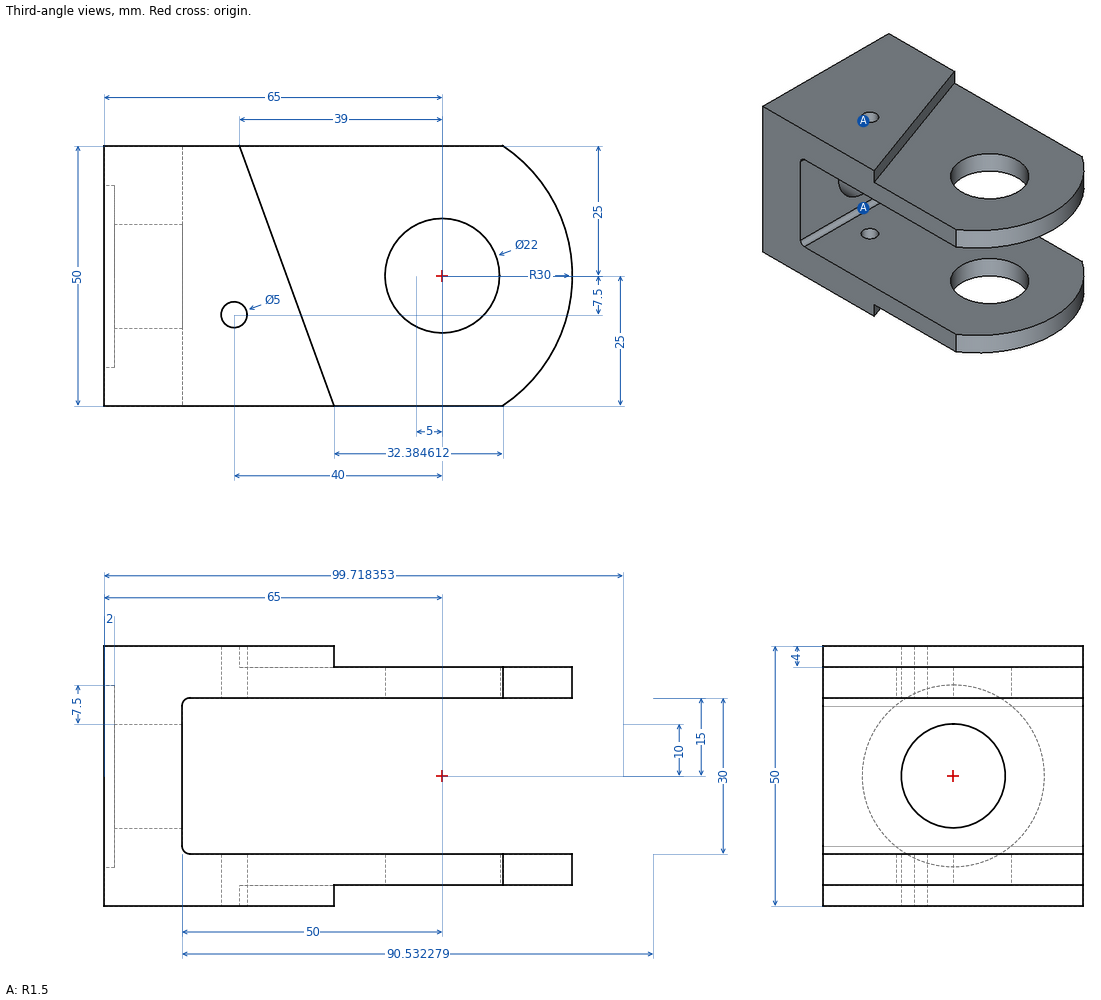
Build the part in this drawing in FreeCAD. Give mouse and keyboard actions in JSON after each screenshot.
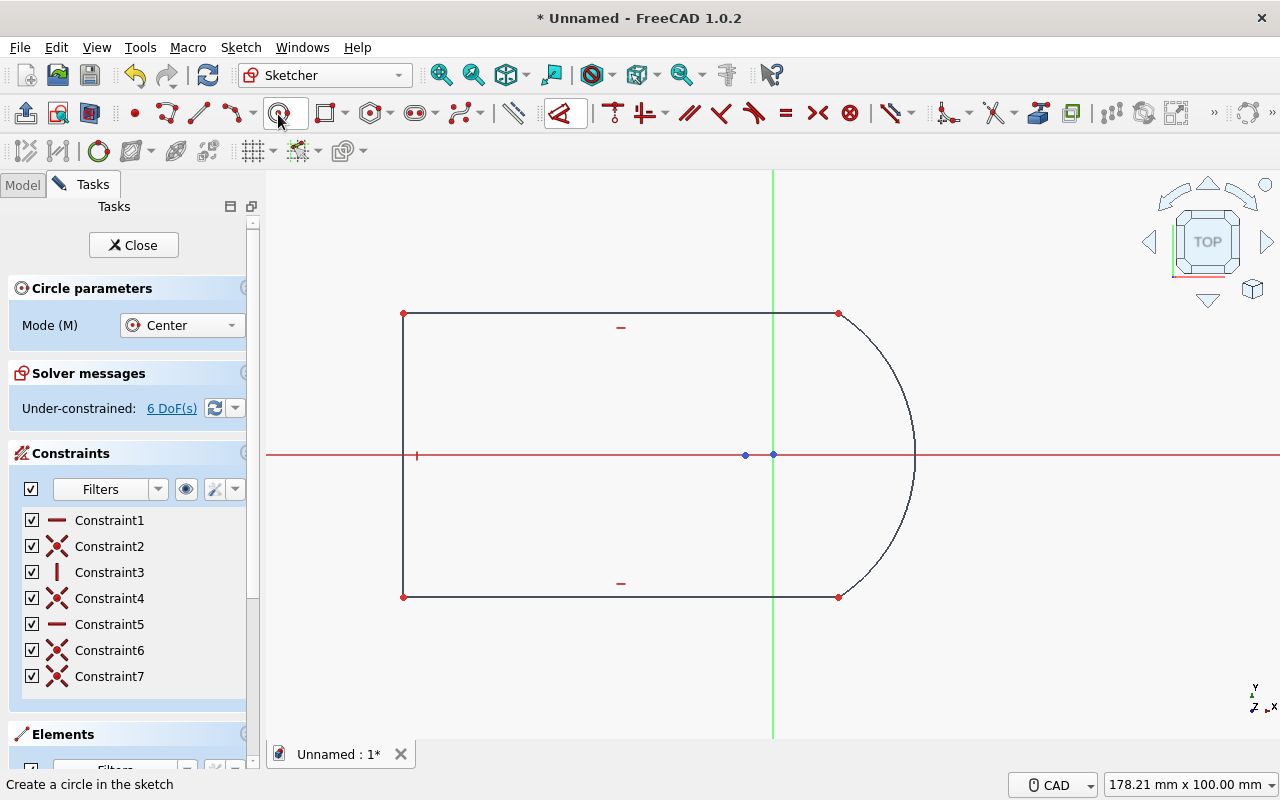
{"action": "scroll", "coordinate": [545, 497], "scroll_direction": "up", "scroll_amount": 3}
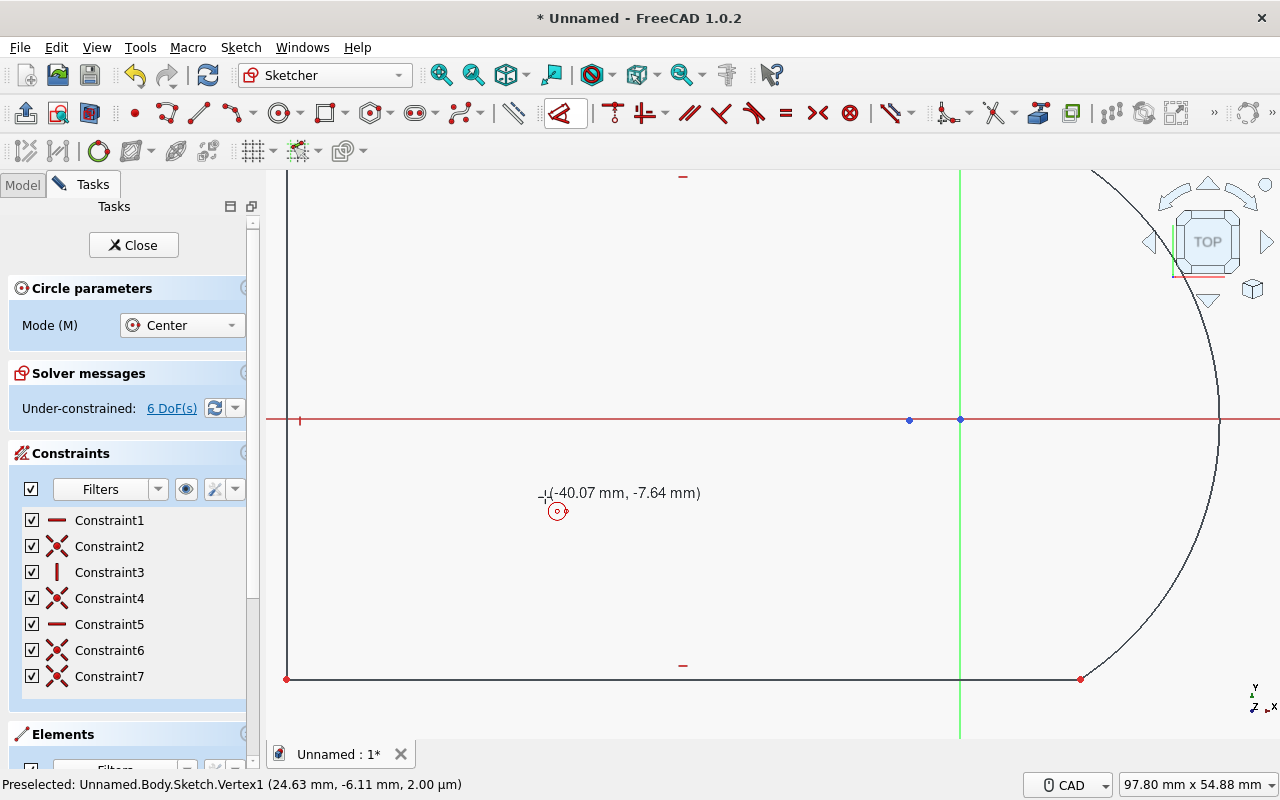
{"action": "left_click", "coordinate": [546, 497]}
{"action": "left_click", "coordinate": [564, 479]}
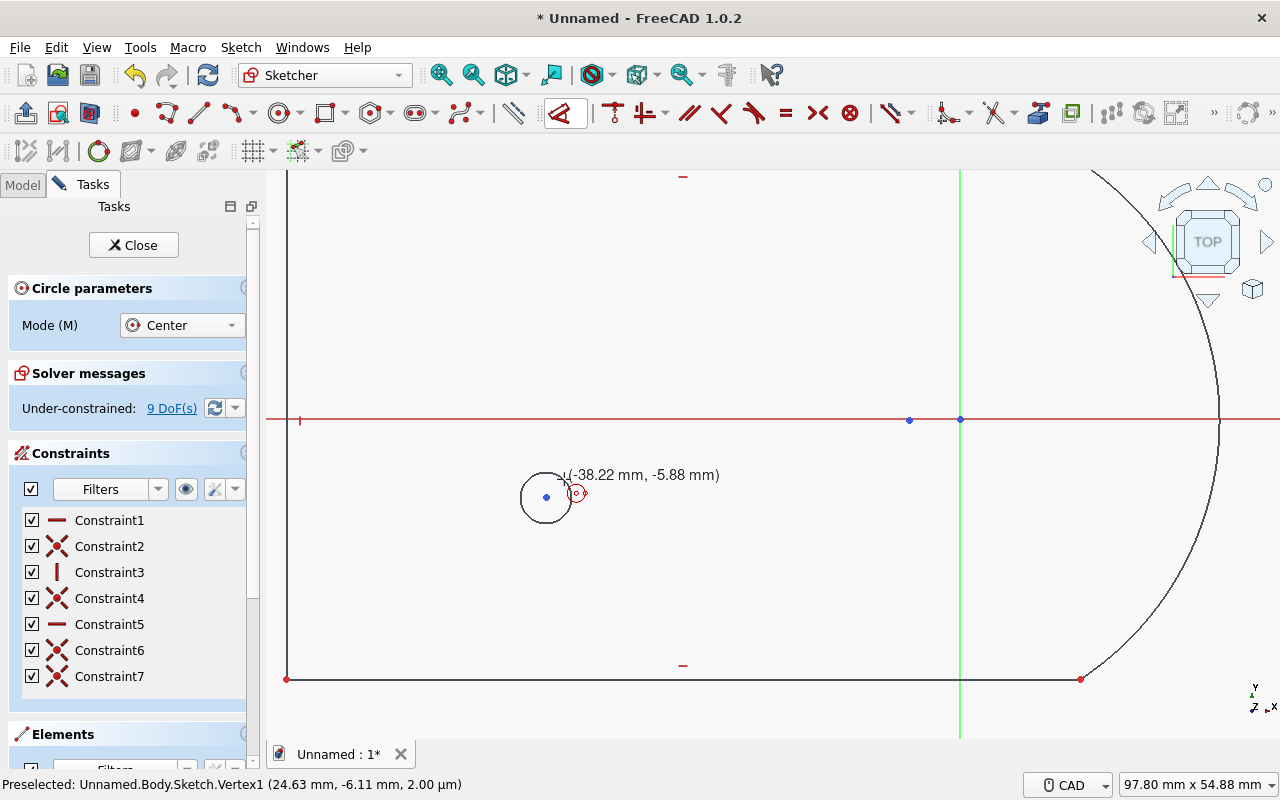
{"action": "left_click", "coordinate": [960, 419]}
{"action": "left_click", "coordinate": [1041, 338]}
{"action": "key", "text": "Escape"}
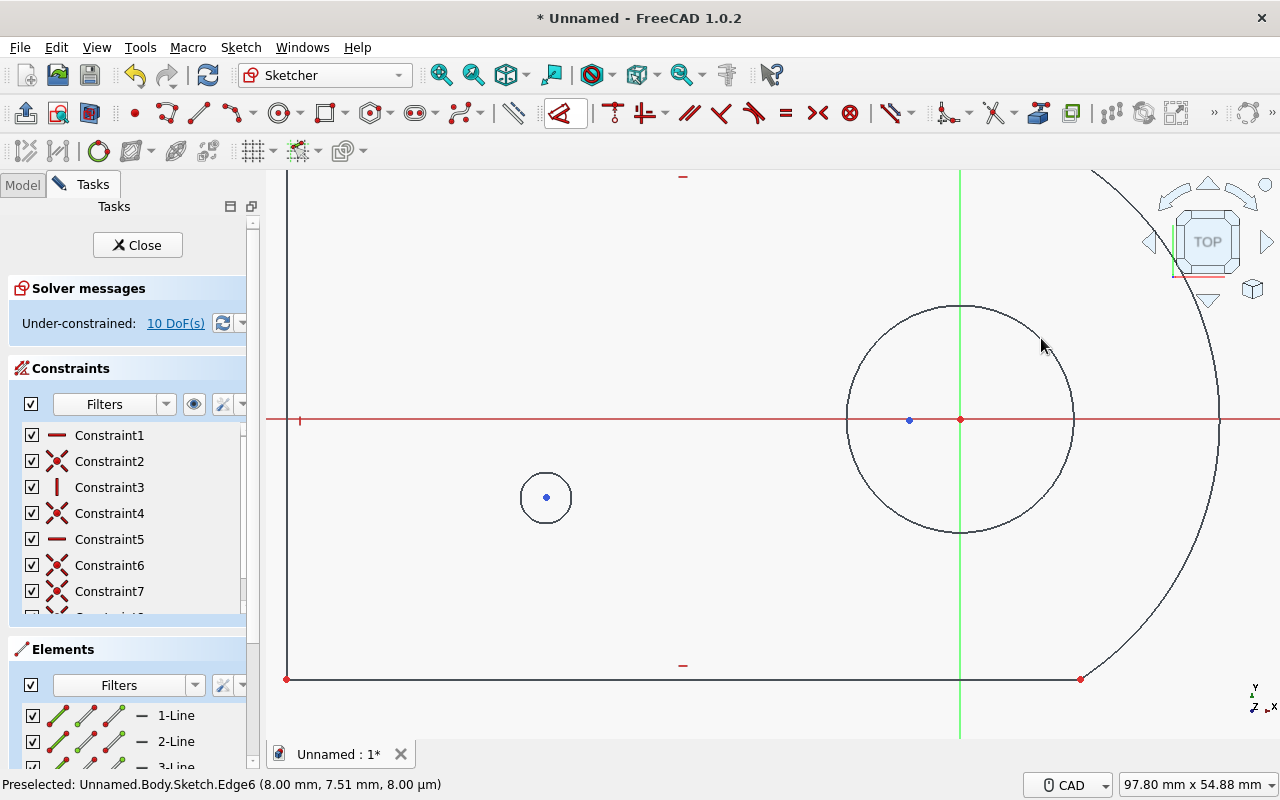
{"action": "left_click", "coordinate": [910, 421]}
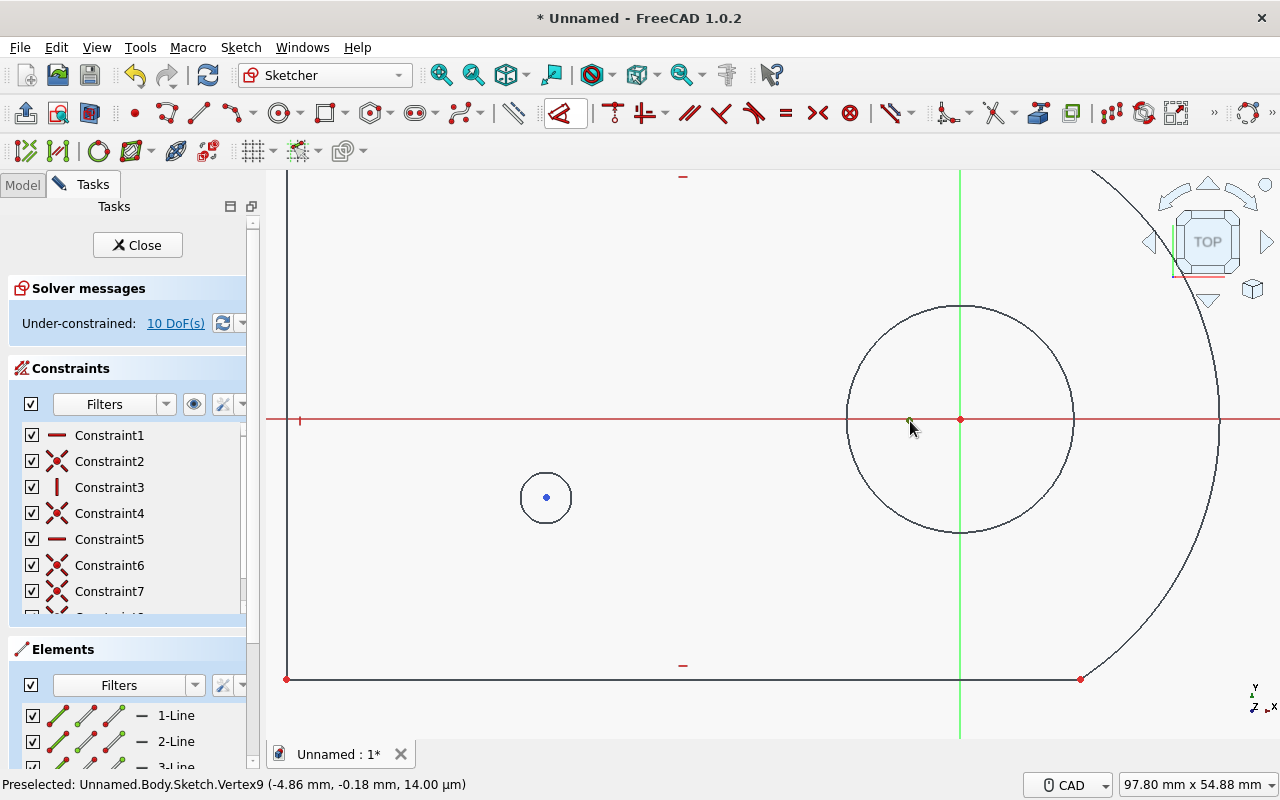
{"action": "left_click", "coordinate": [353, 419]}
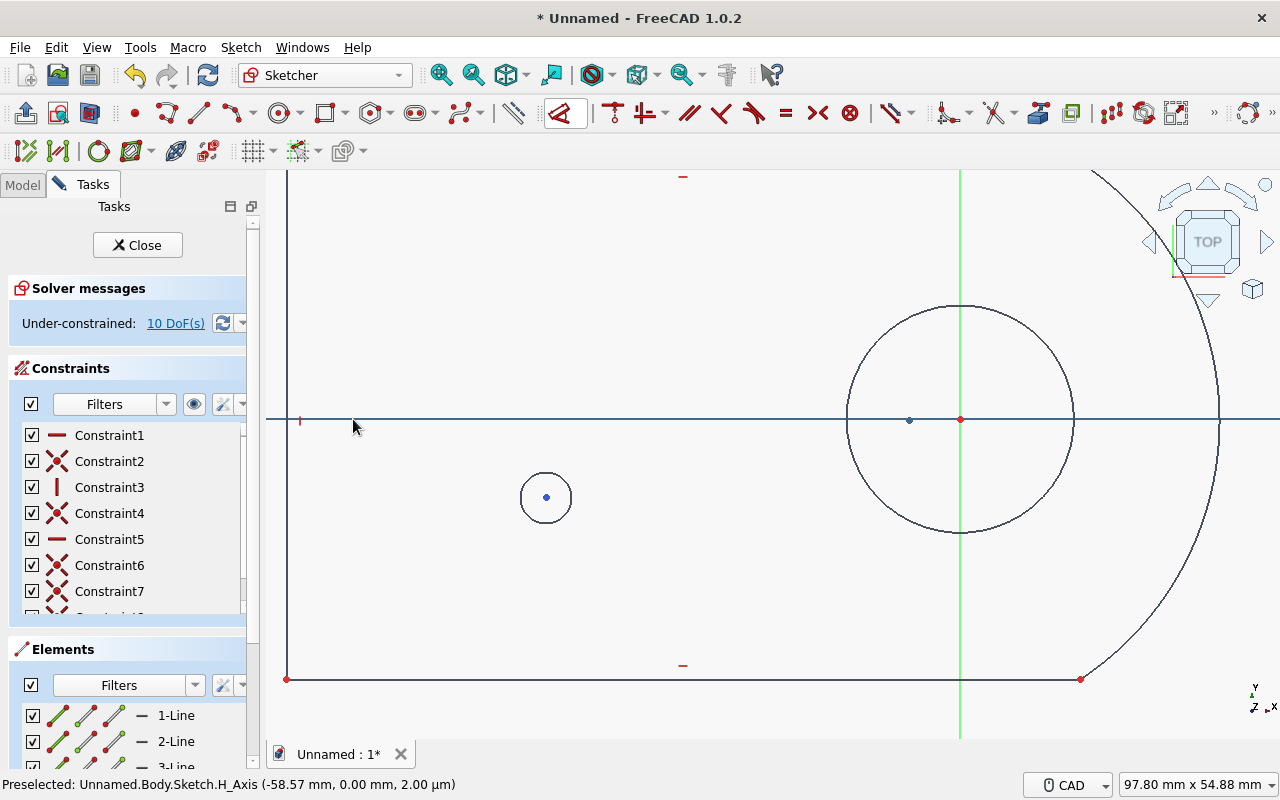
{"action": "left_click", "coordinate": [614, 114]}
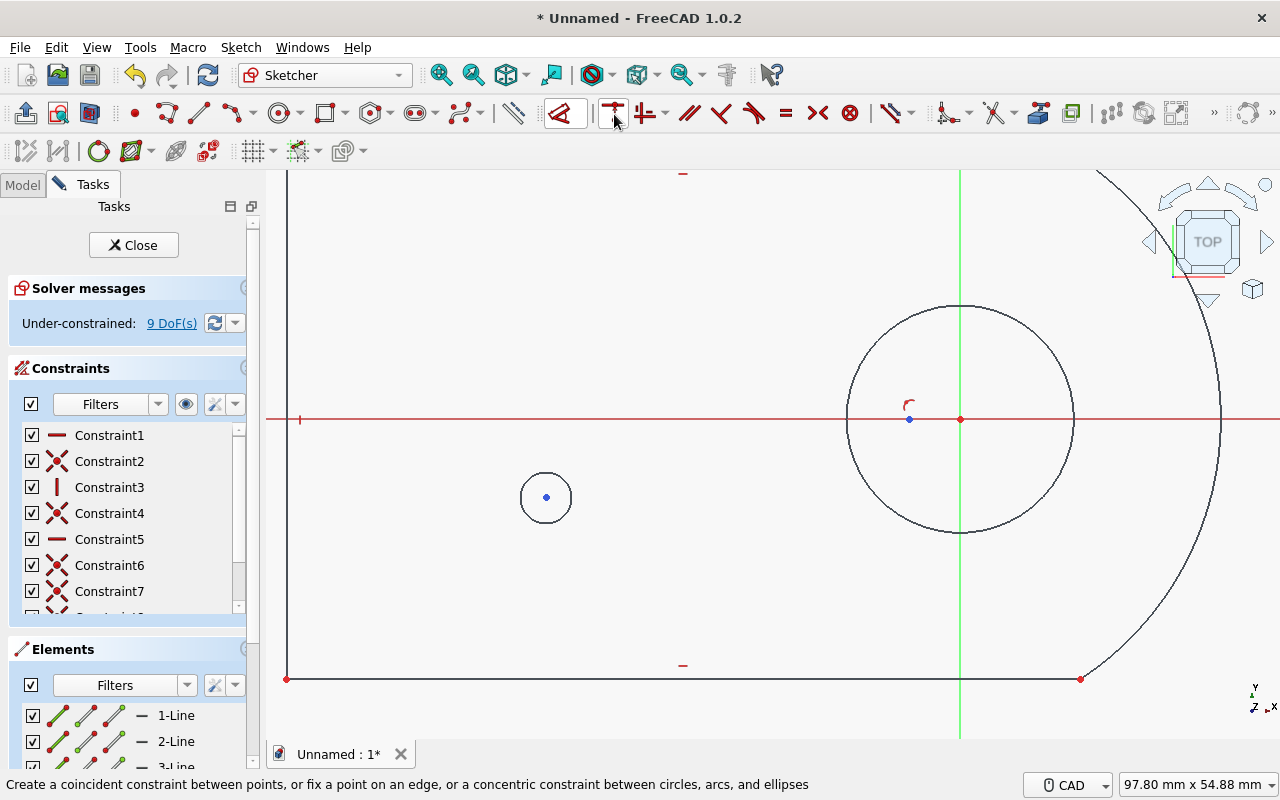
{"action": "left_click", "coordinate": [560, 114]}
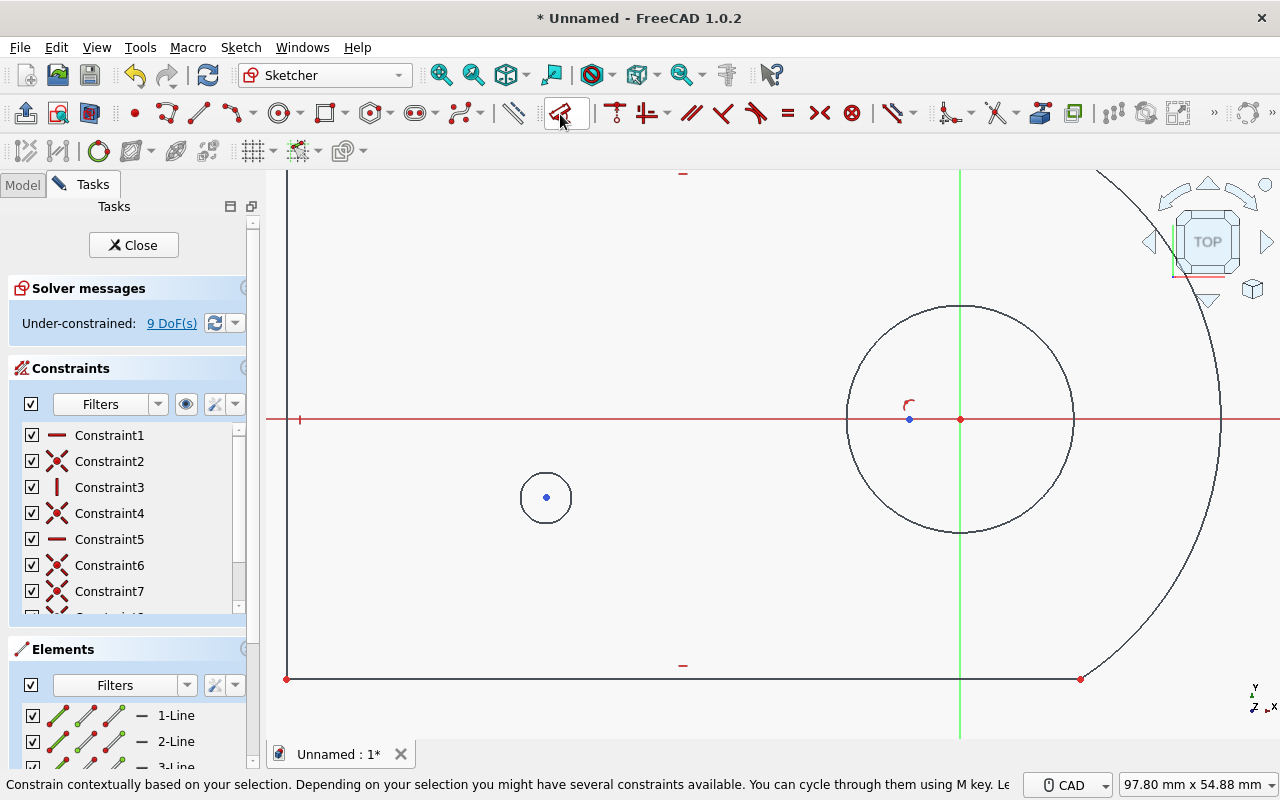
{"action": "scroll", "coordinate": [606, 527], "scroll_direction": "down", "scroll_amount": 2}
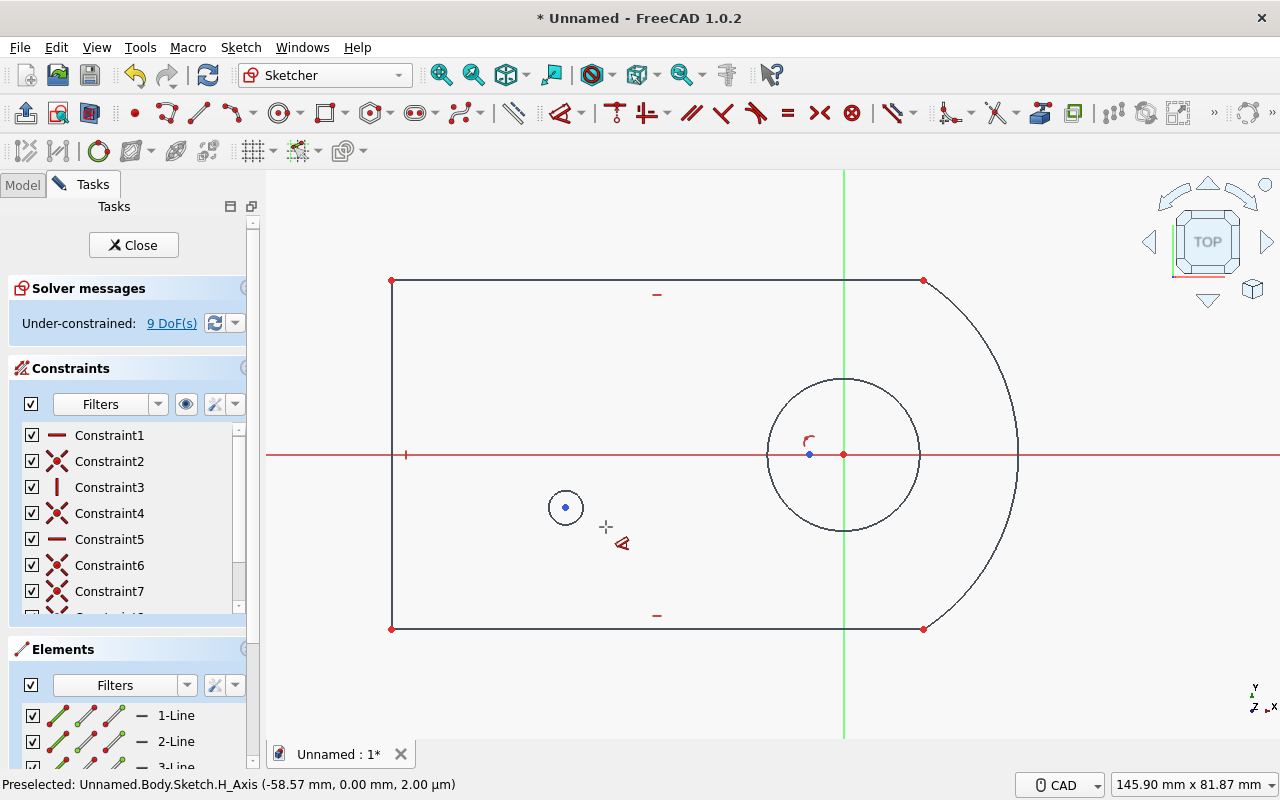
{"action": "left_click", "coordinate": [1002, 535]}
{"action": "left_click", "coordinate": [1032, 547]}